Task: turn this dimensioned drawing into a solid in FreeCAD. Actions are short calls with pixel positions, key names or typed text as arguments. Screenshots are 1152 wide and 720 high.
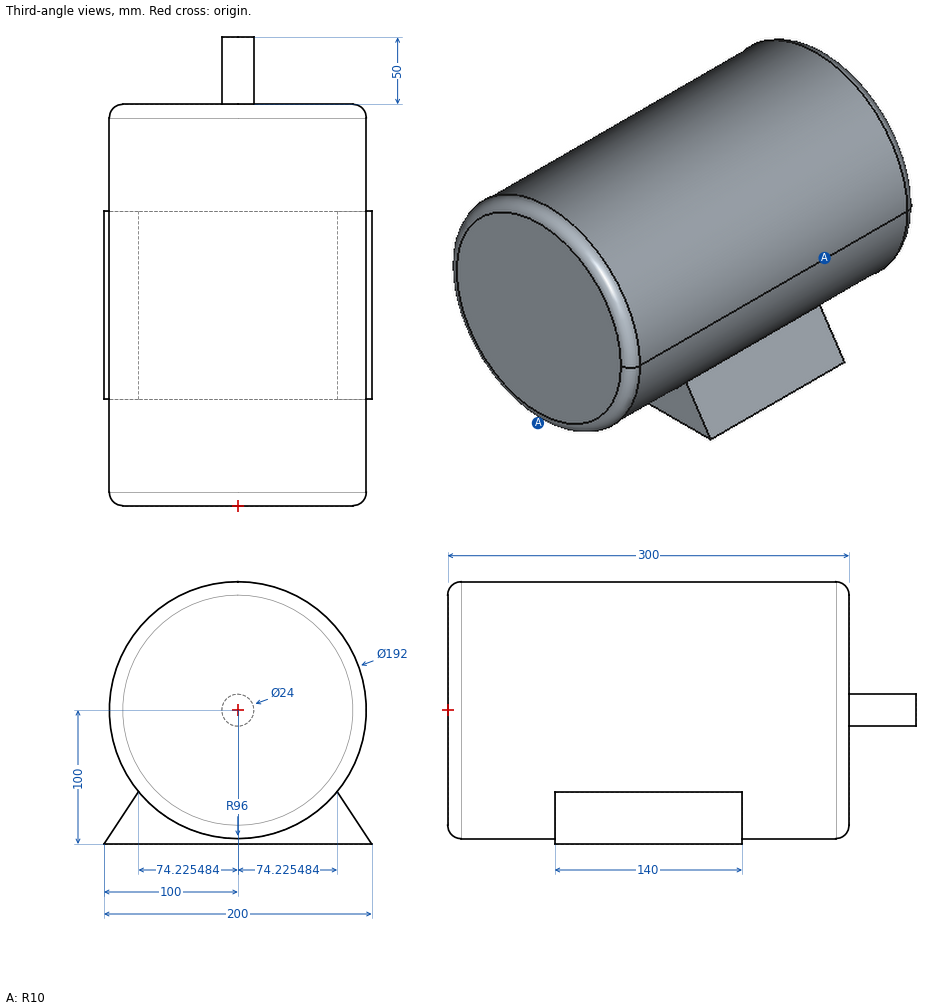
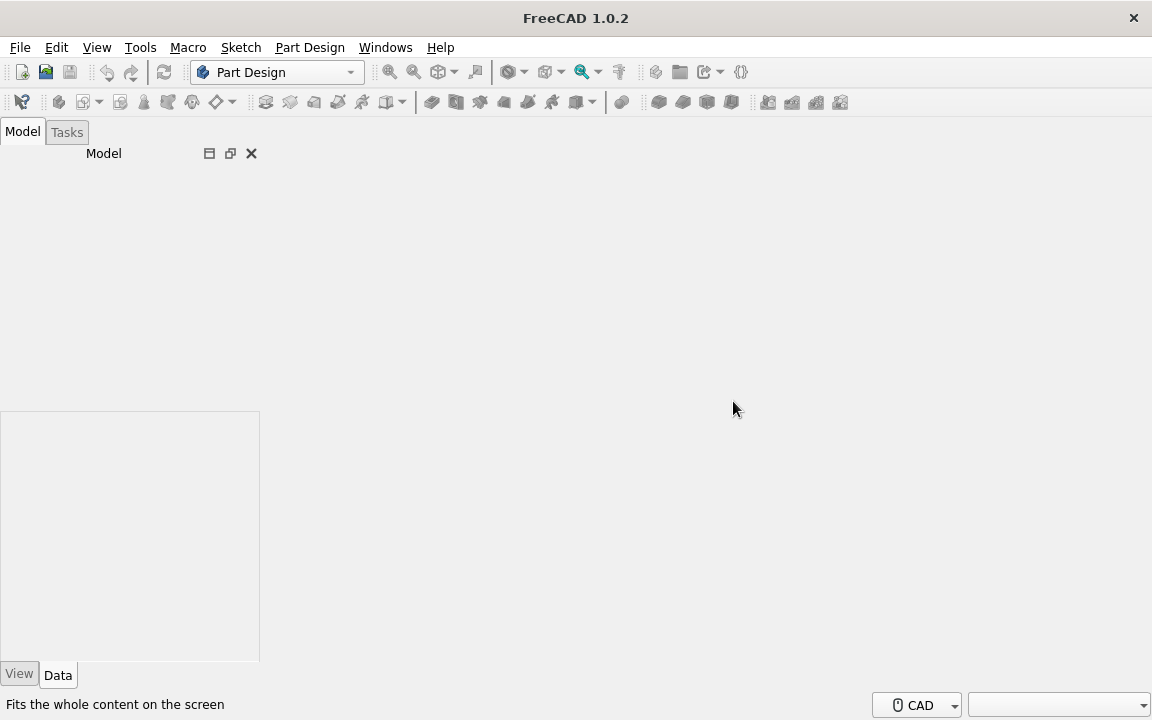
click(22, 72)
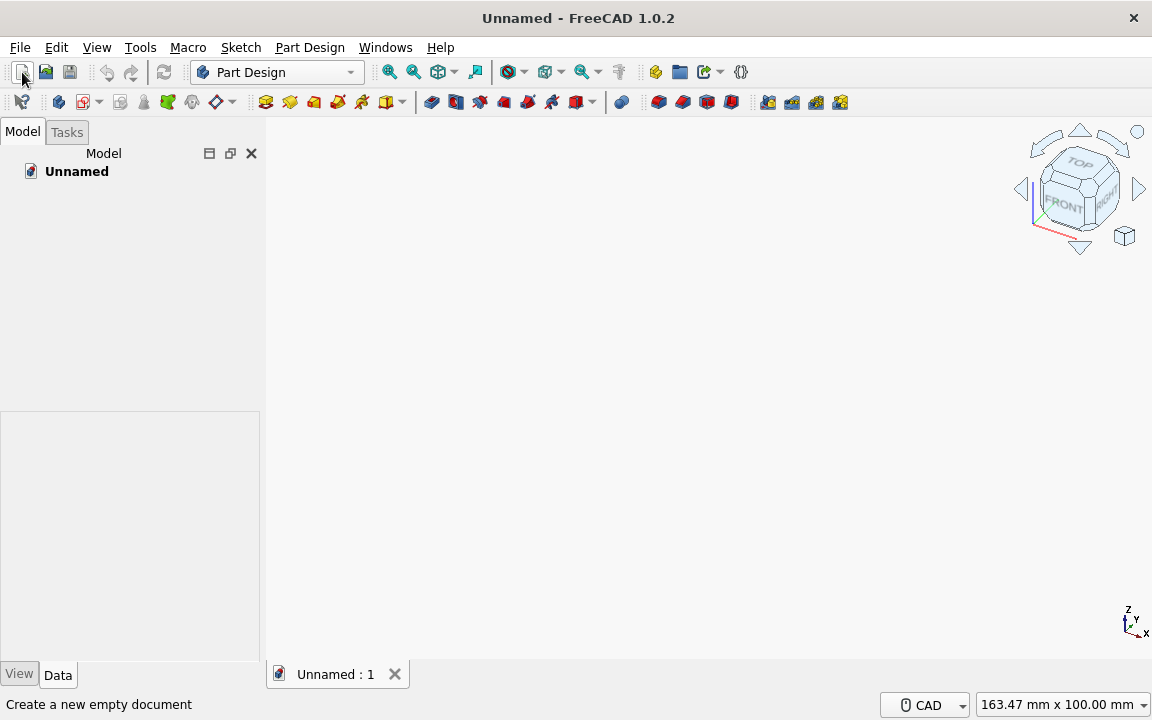
click(84, 102)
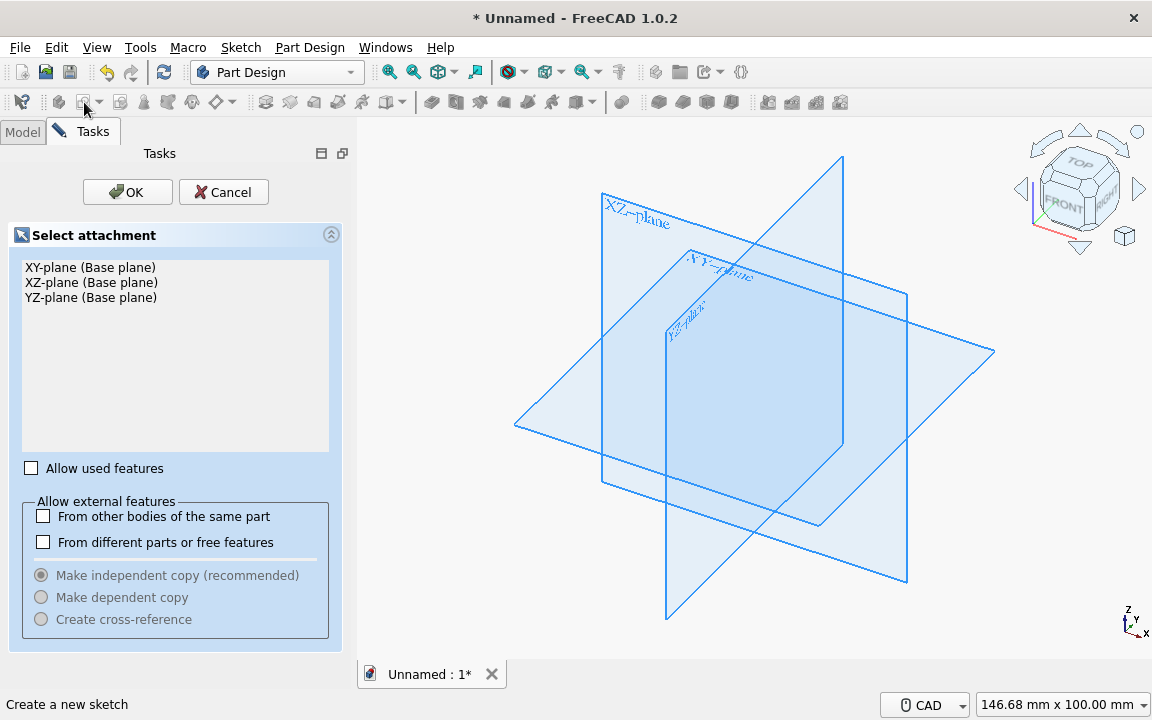
click(82, 282)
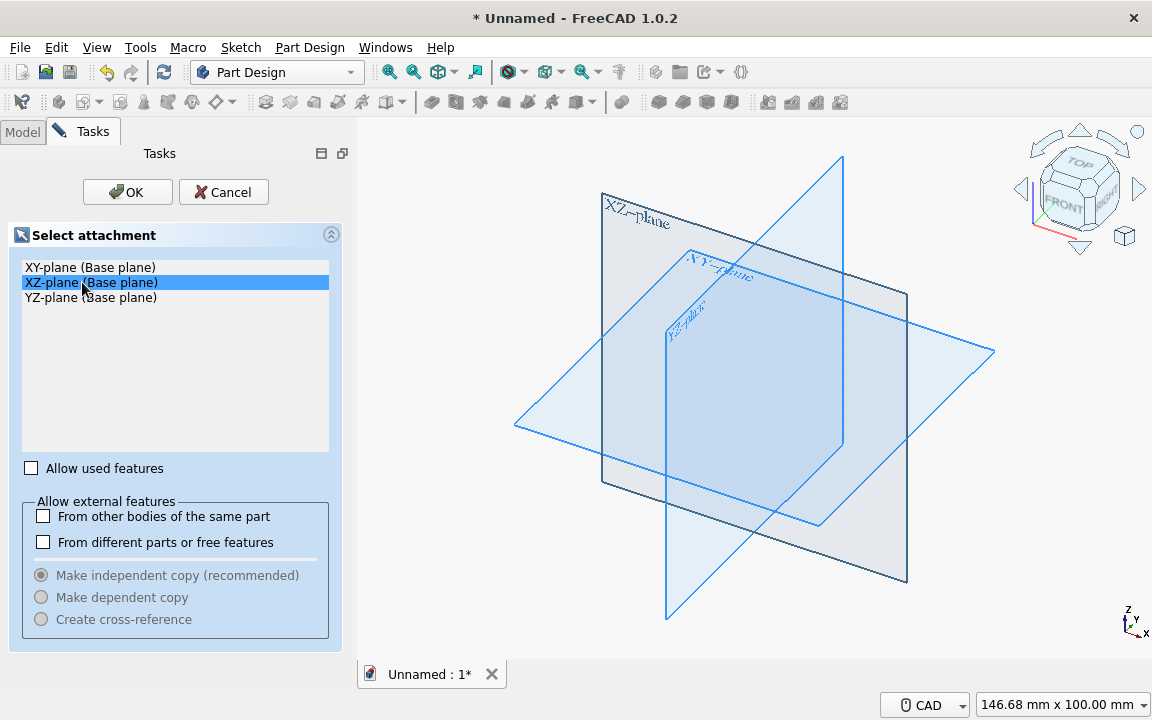
click(128, 192)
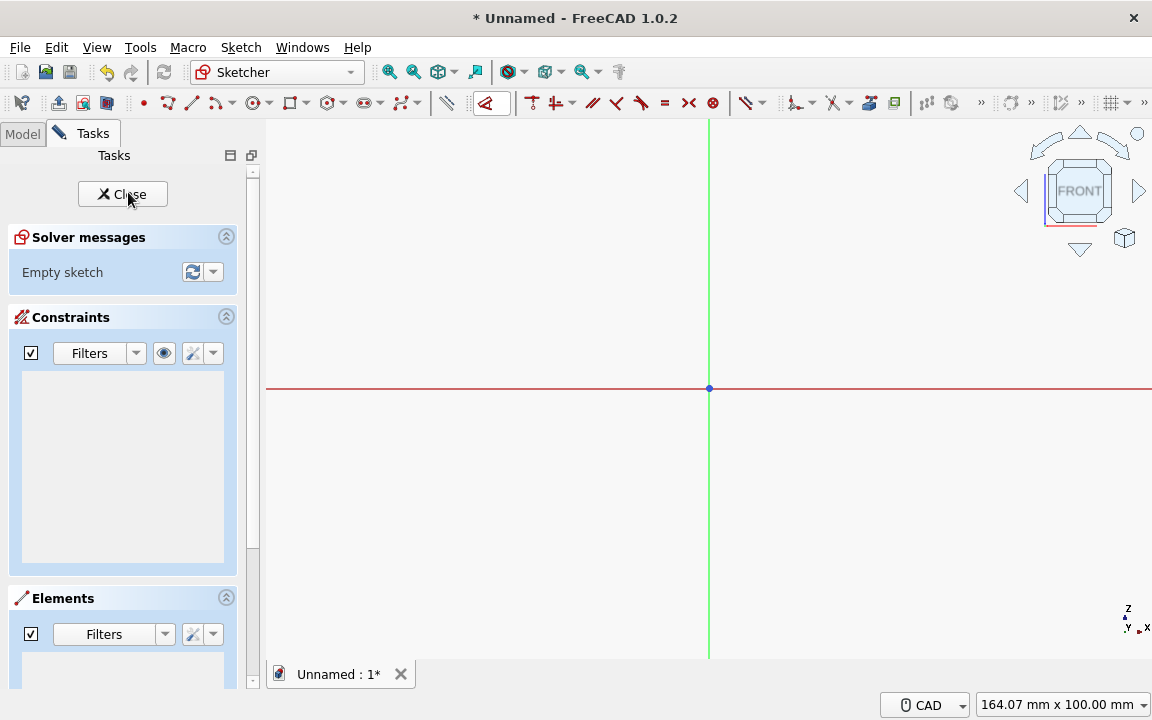
scroll(611, 389, down, 6)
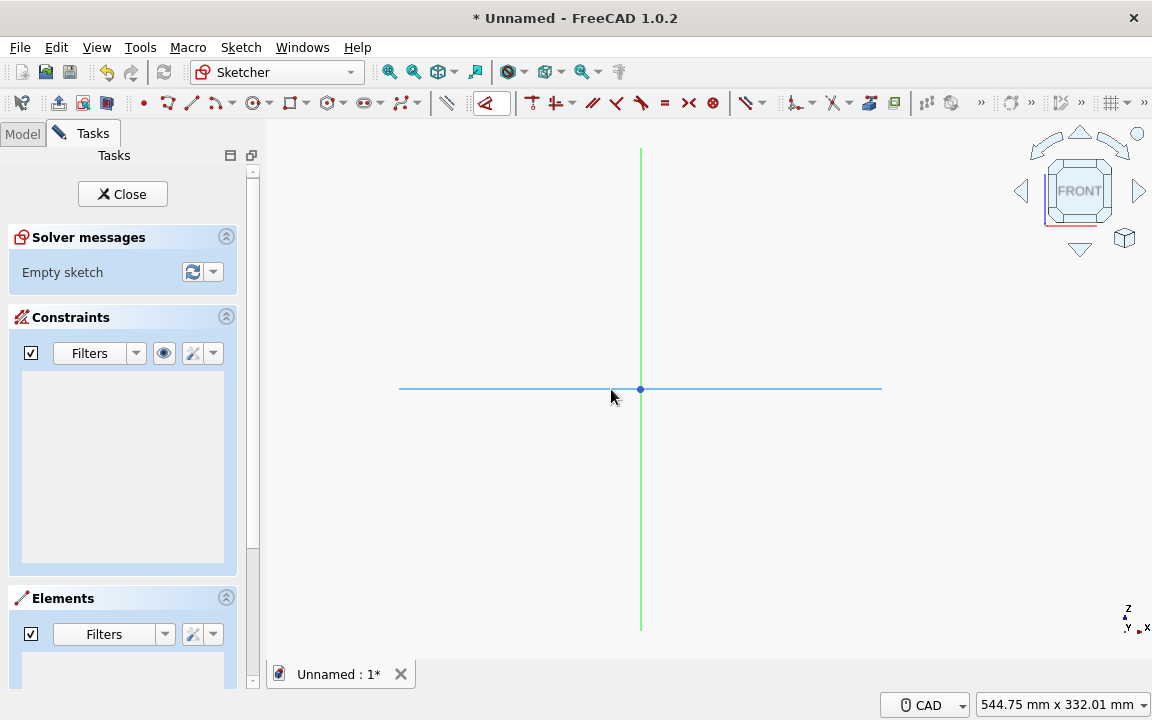
click(254, 104)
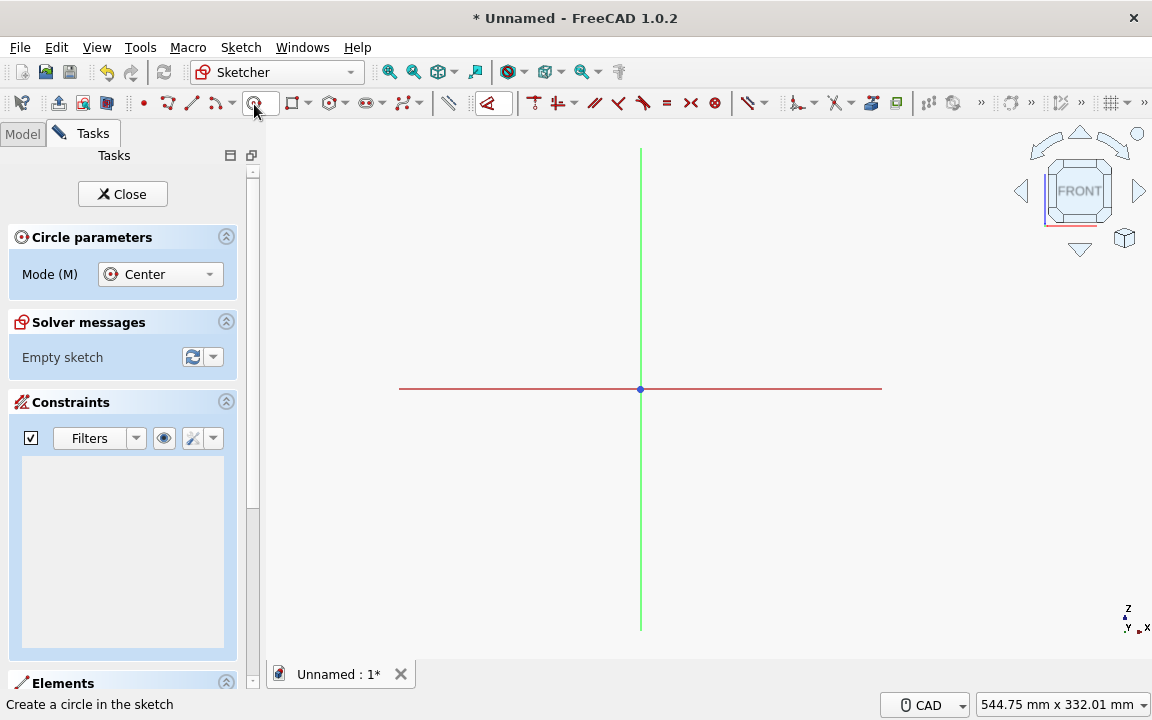
click(641, 389)
move(751, 279)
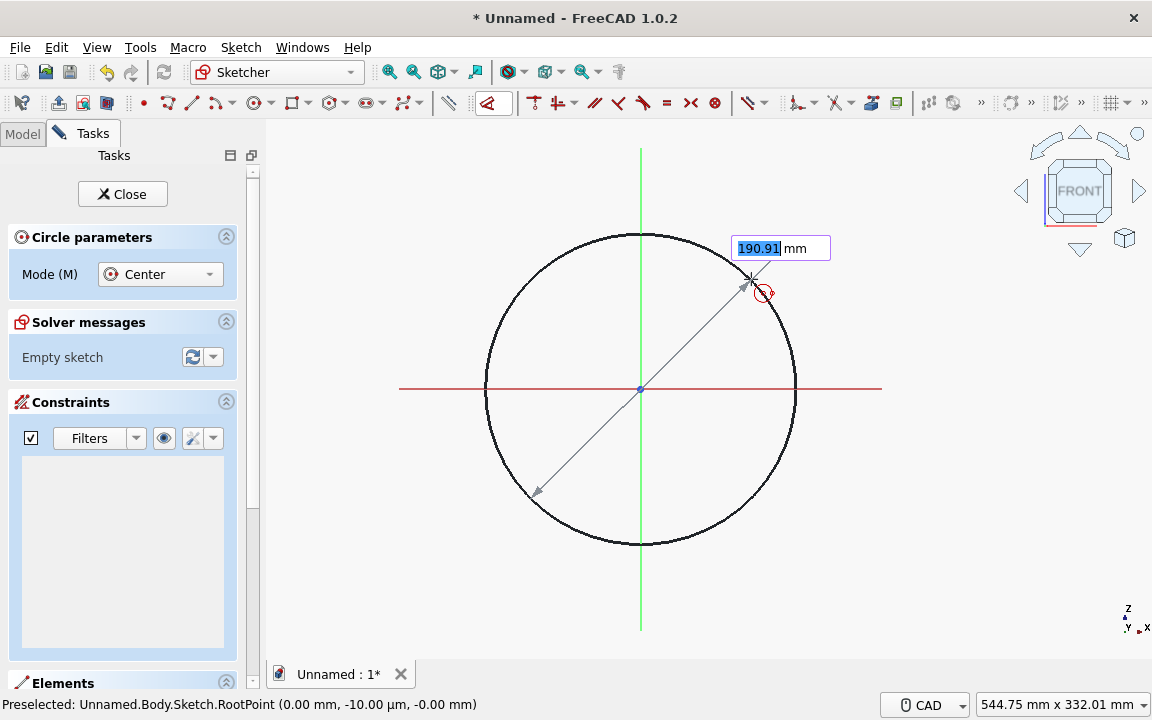
text(192)
key(Return)
key(Escape)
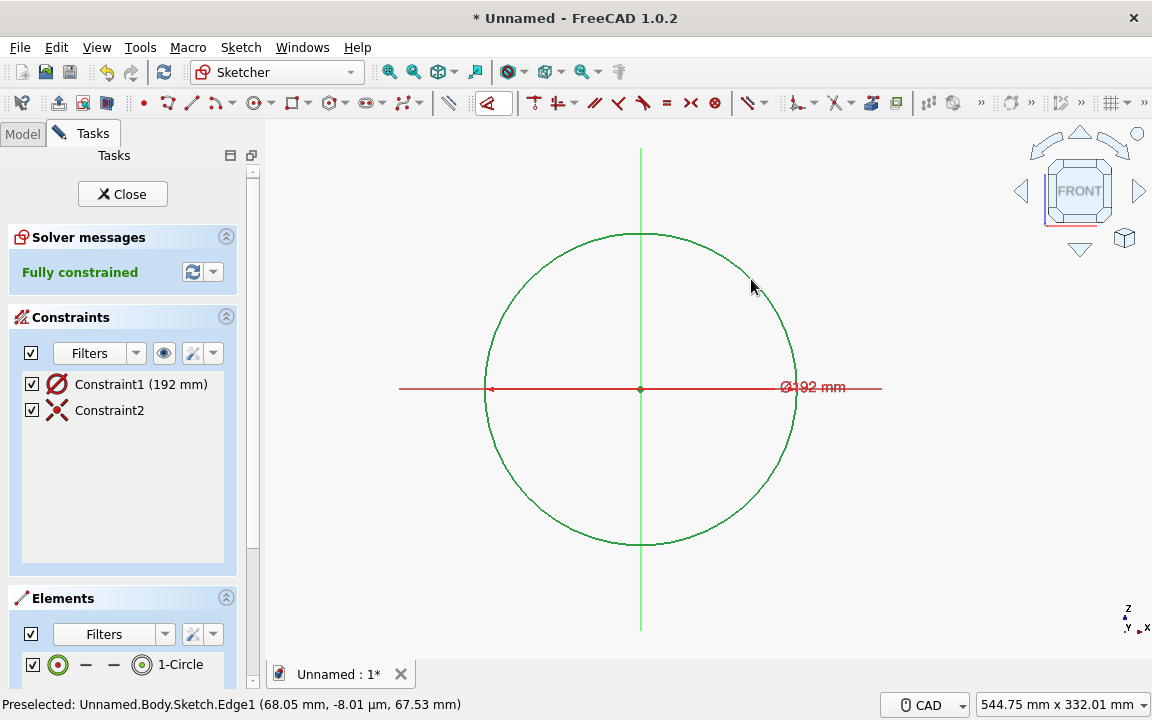
click(123, 194)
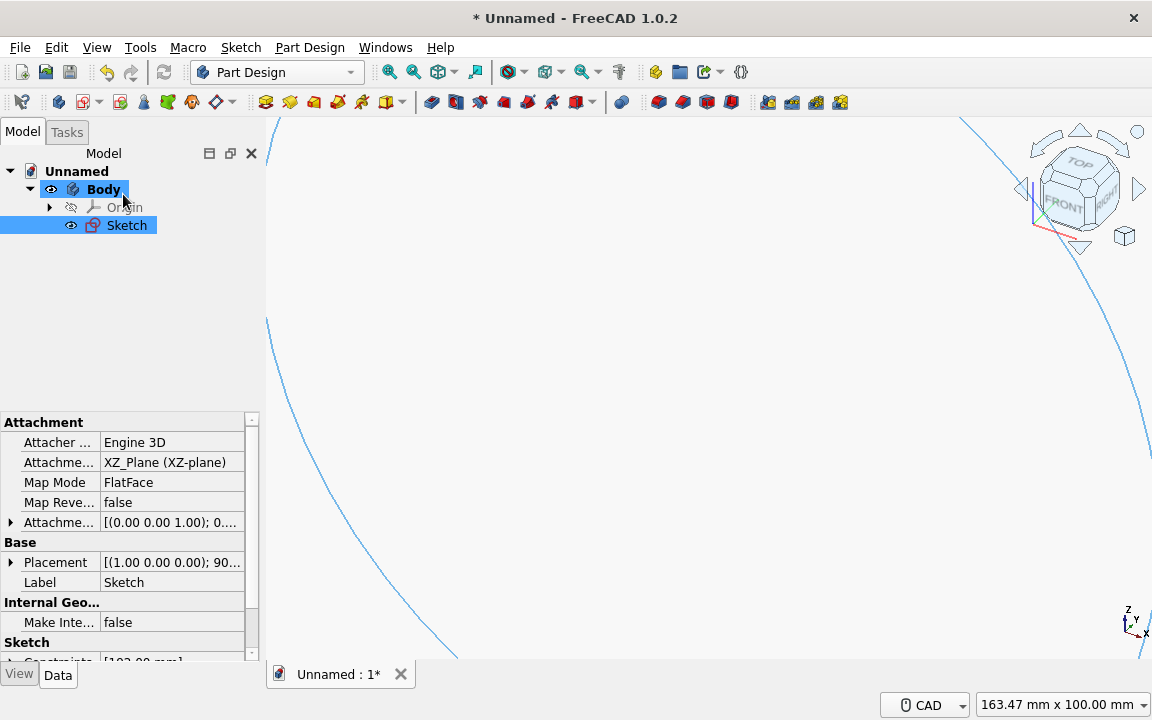
click(266, 102)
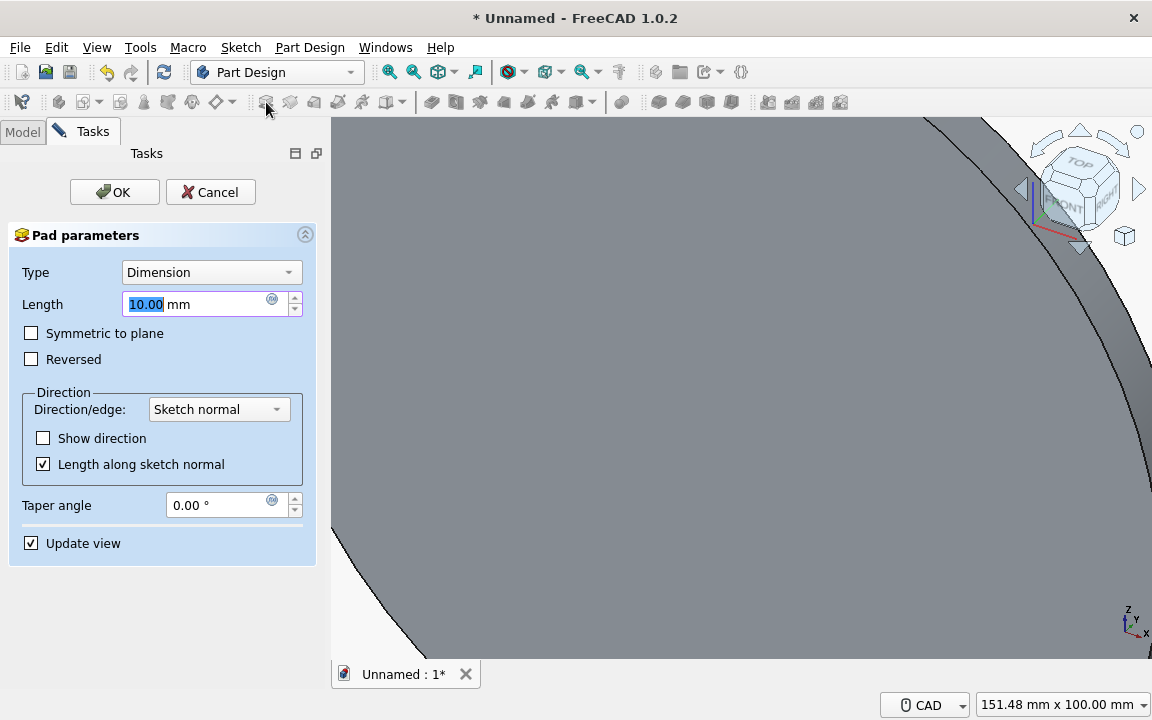
text(300)
key(Tab)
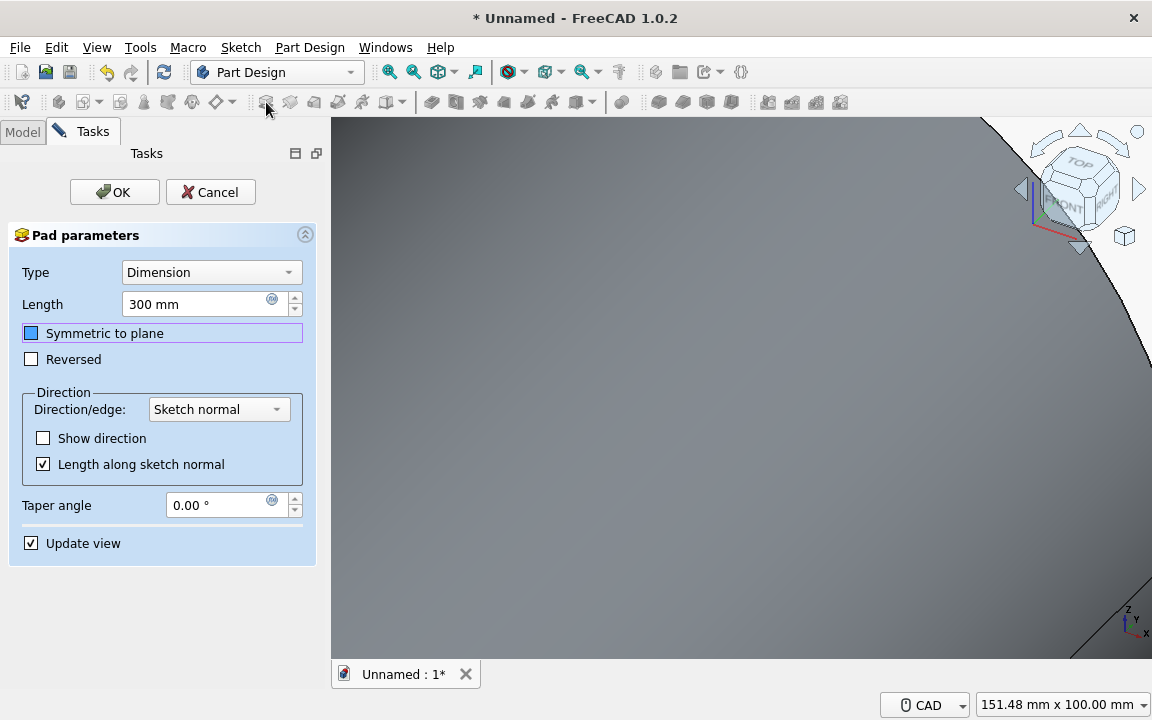
click(30, 359)